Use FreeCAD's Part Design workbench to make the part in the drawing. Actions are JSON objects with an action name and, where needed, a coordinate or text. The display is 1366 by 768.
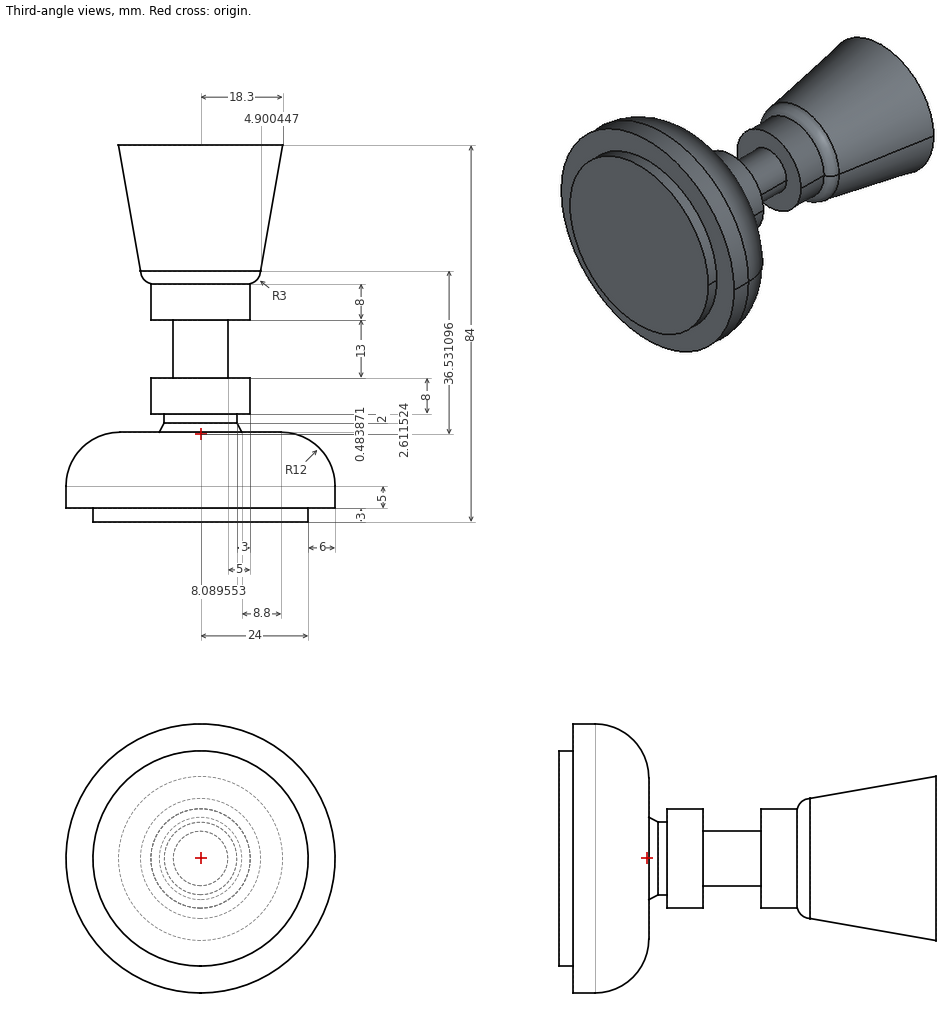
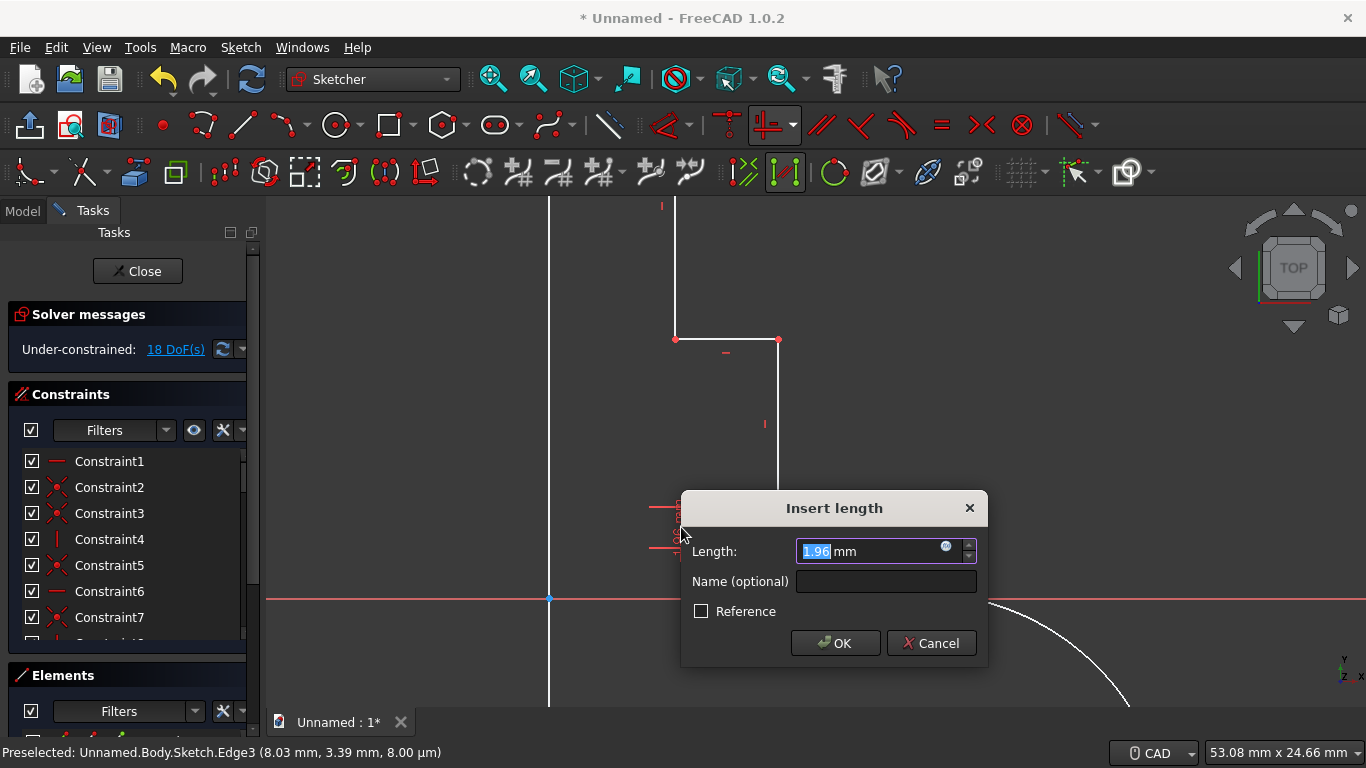
{"action": "type", "text": "2"}
{"action": "key", "text": "Return"}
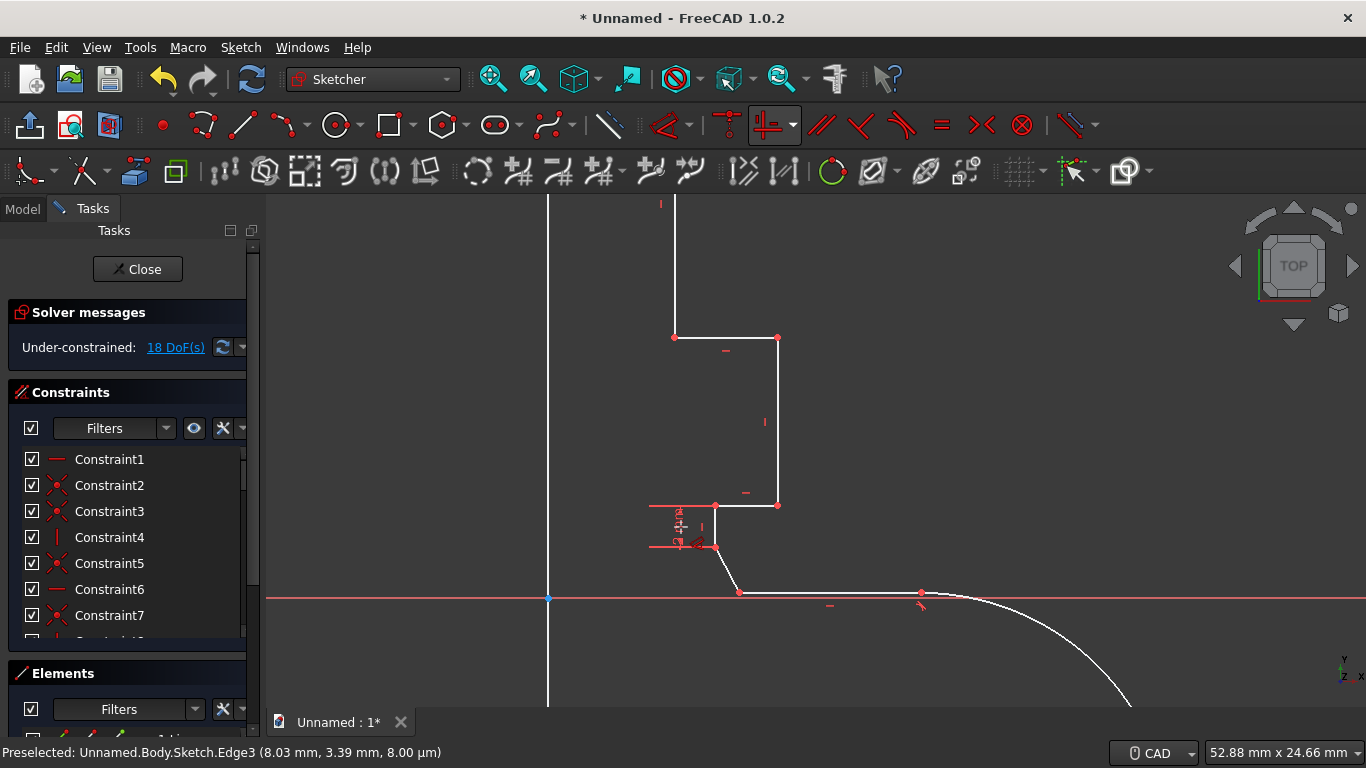
{"action": "left_click", "coordinate": [734, 506]}
{"action": "left_click", "coordinate": [761, 540]}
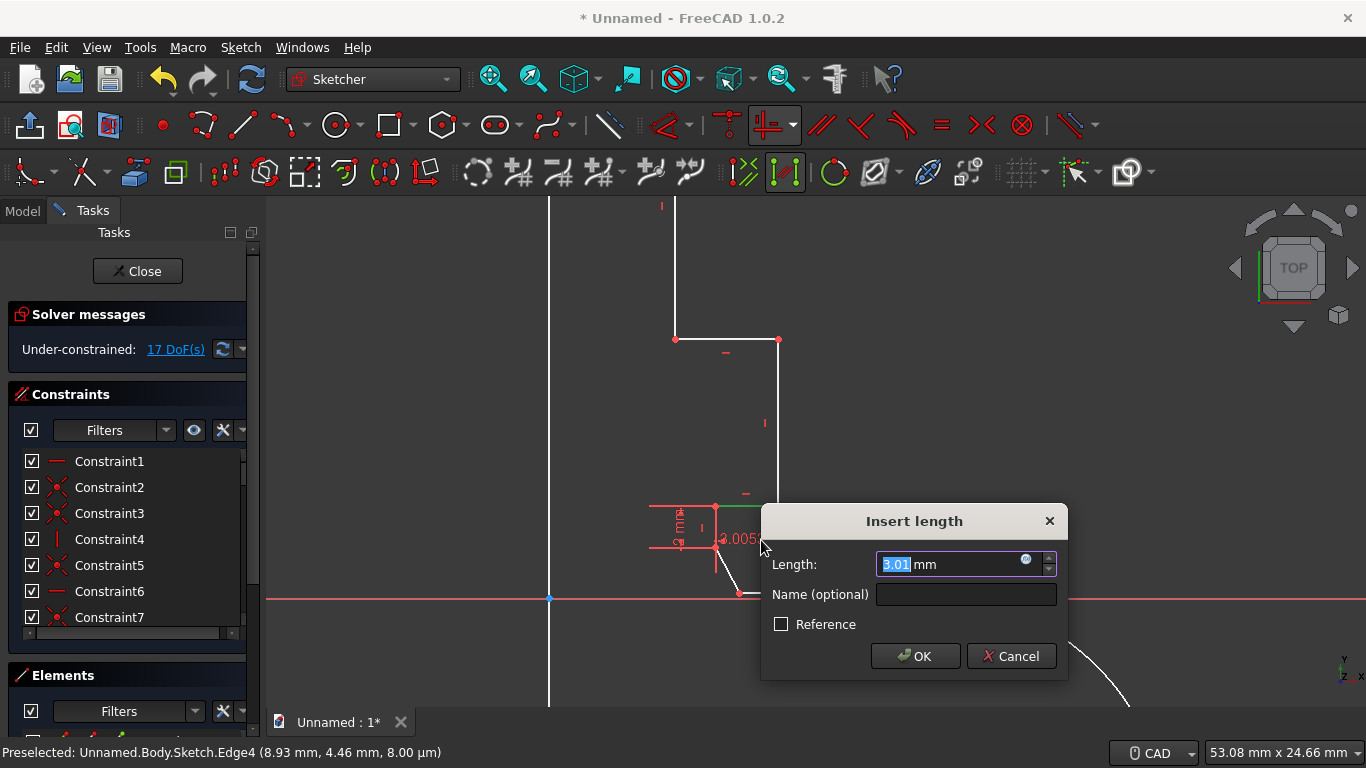
{"action": "type", "text": "3"}
{"action": "key", "text": "Return"}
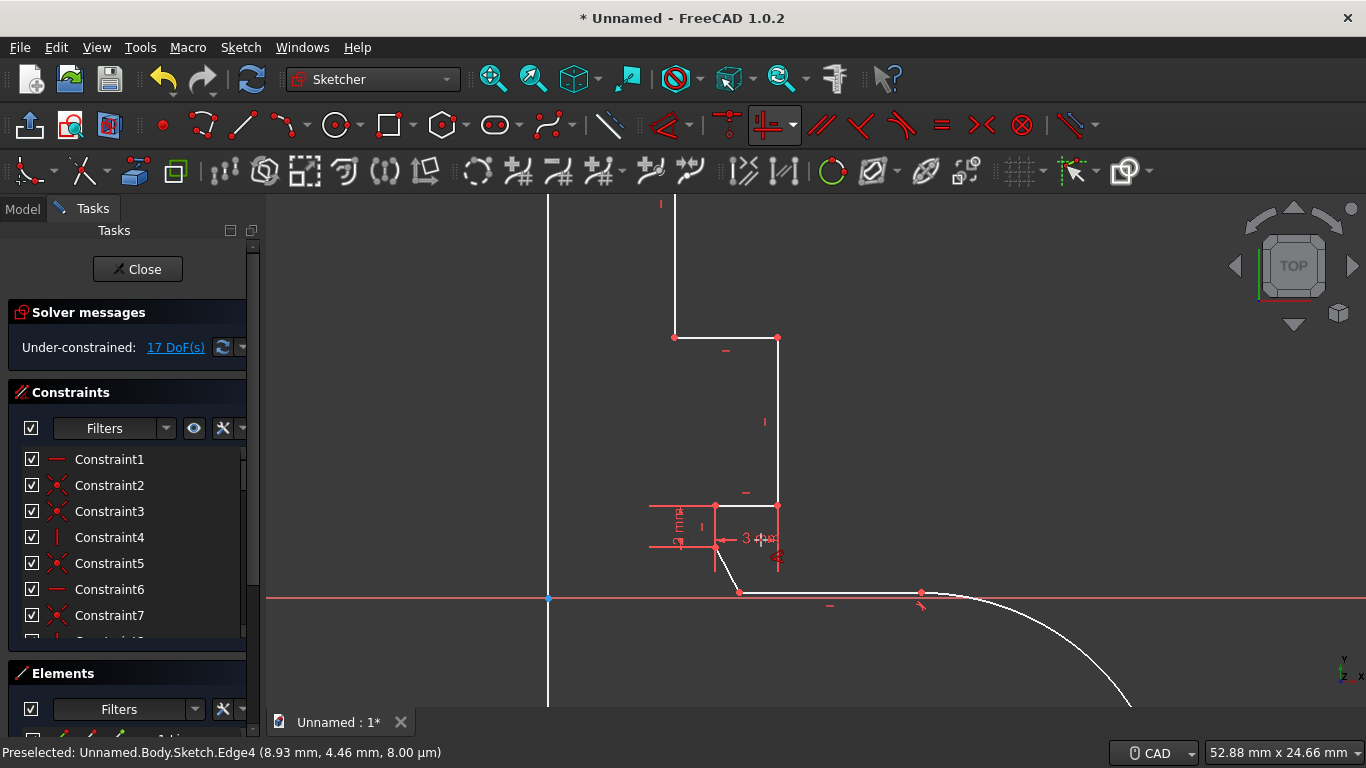
{"action": "scroll", "coordinate": [719, 531], "scroll_direction": "down", "scroll_amount": 8}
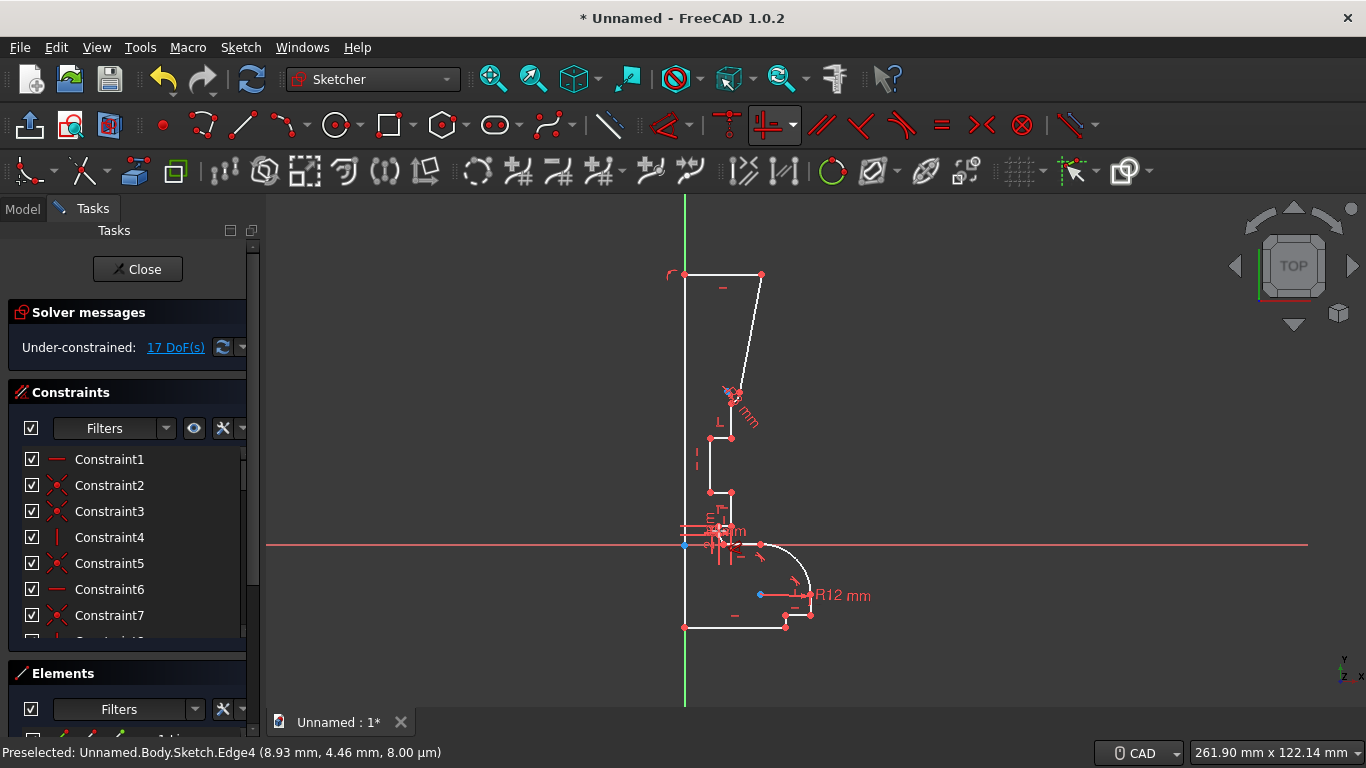
{"action": "scroll", "coordinate": [731, 516], "scroll_direction": "up", "scroll_amount": 2}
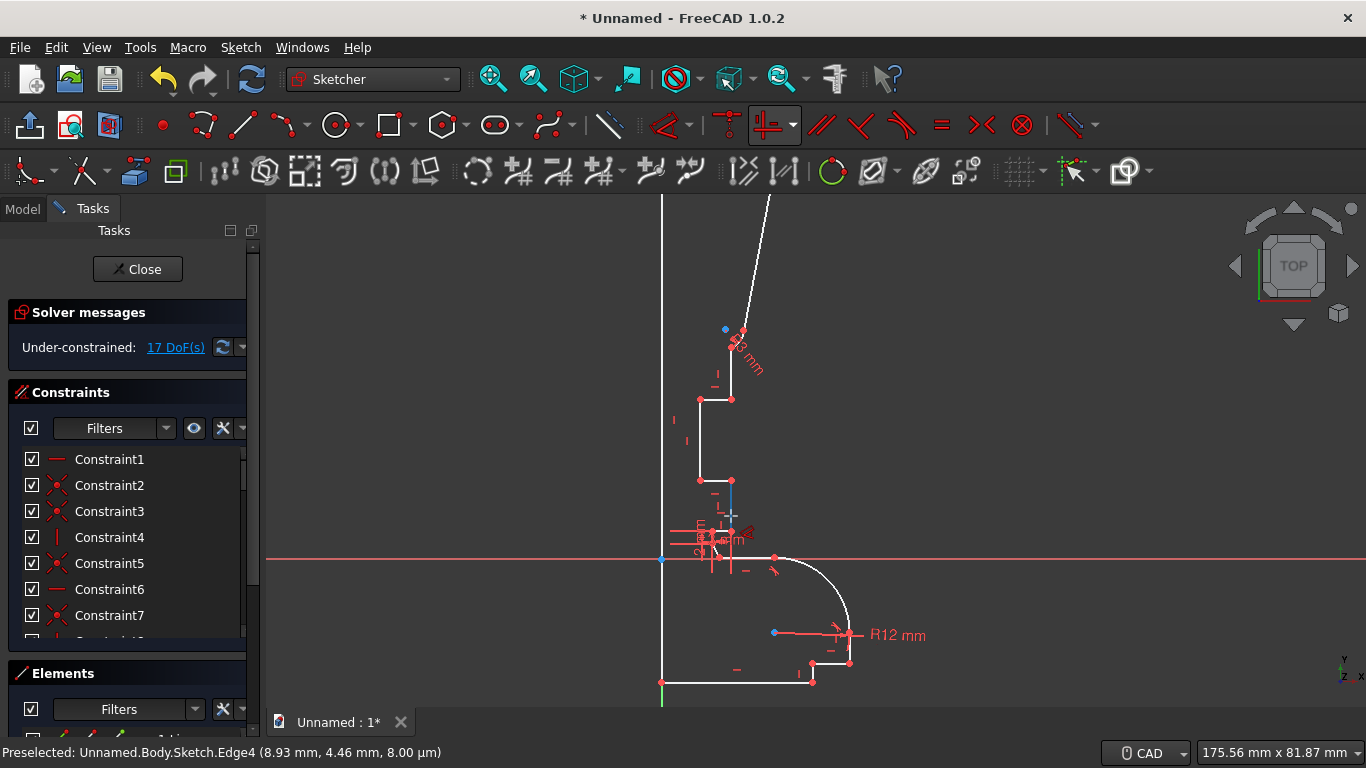
{"action": "left_click", "coordinate": [731, 516]}
{"action": "left_click", "coordinate": [697, 506]}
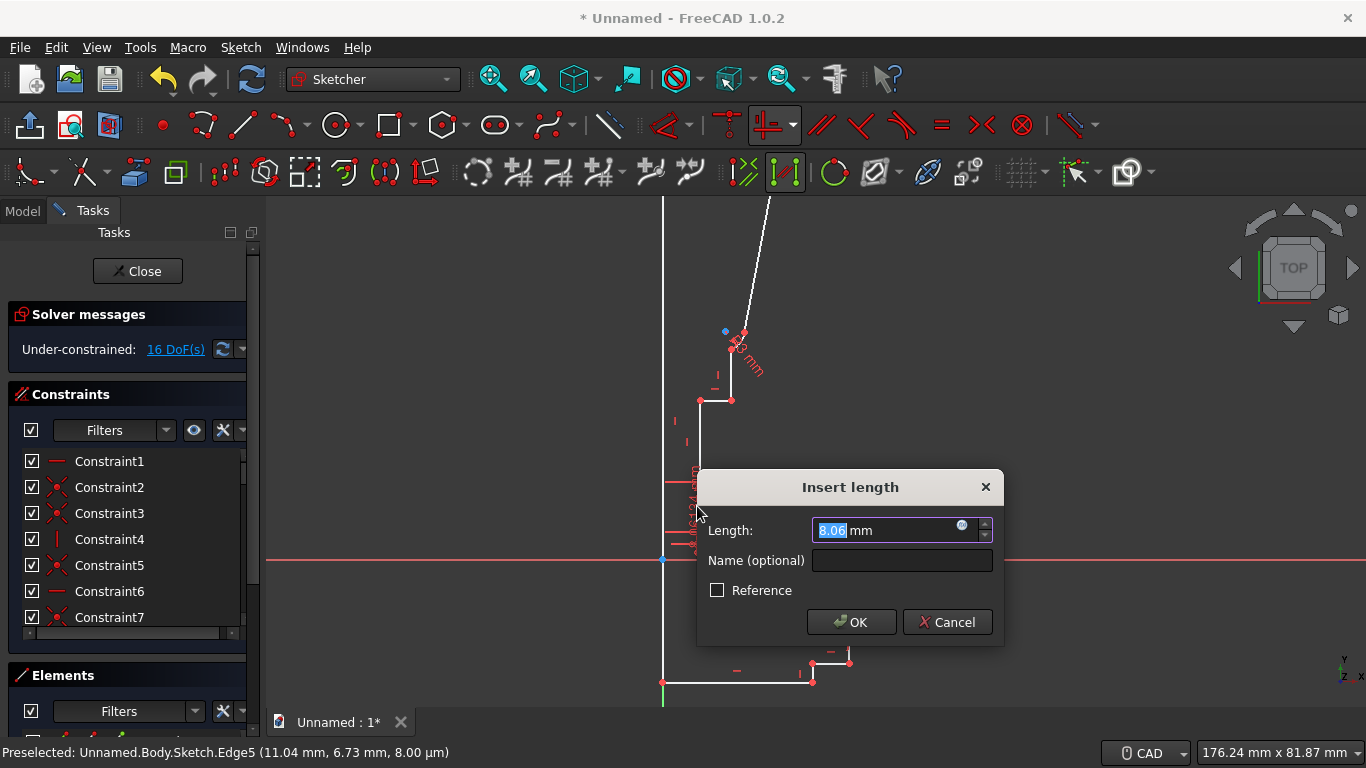
{"action": "type", "text": "8"}
{"action": "key", "text": "Return"}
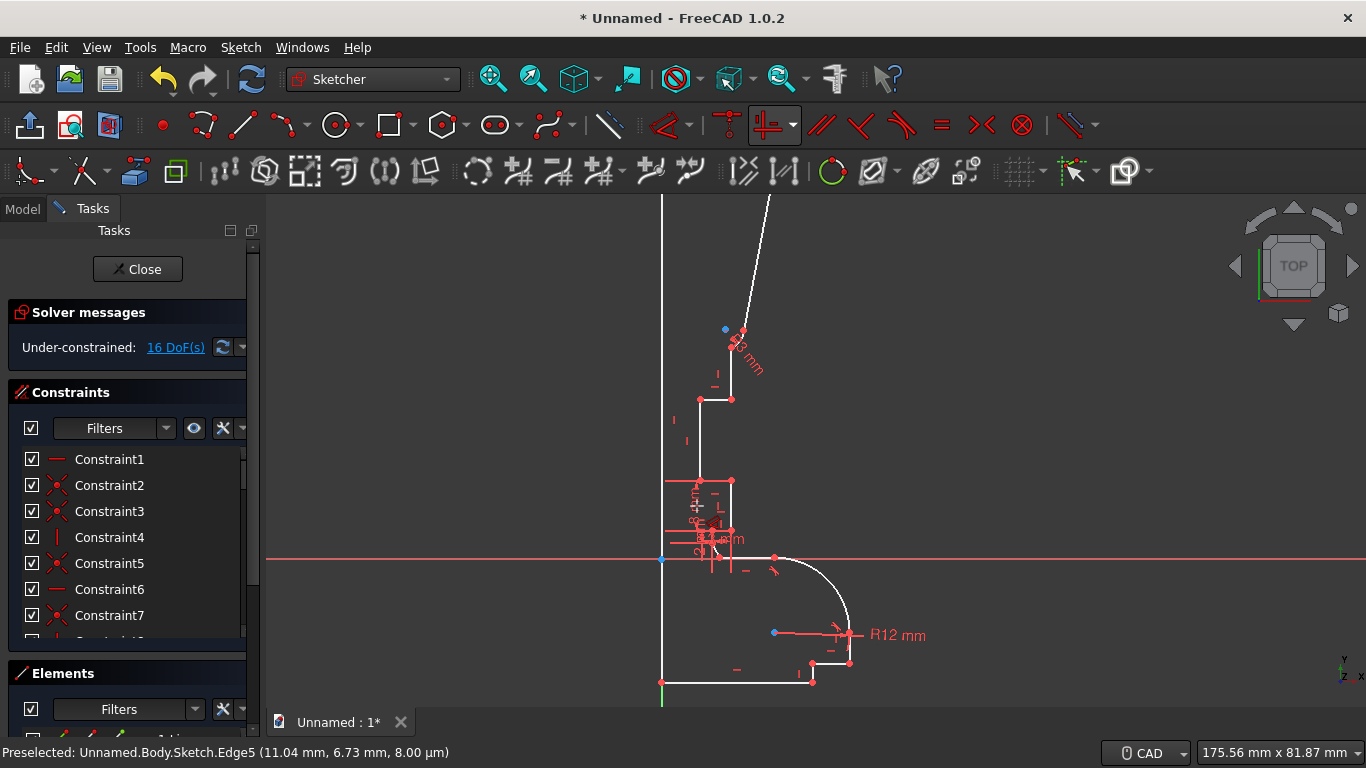
{"action": "scroll", "coordinate": [722, 481], "scroll_direction": "up", "scroll_amount": 2}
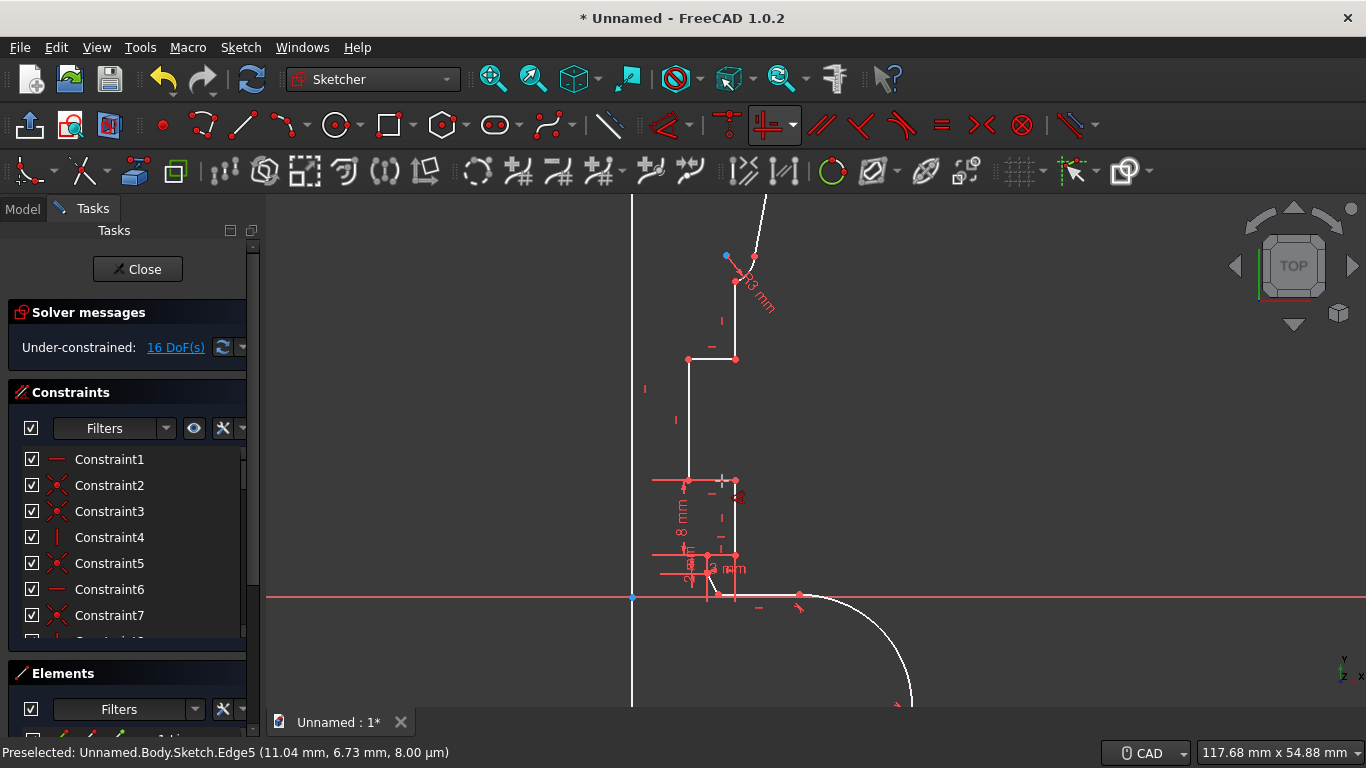
{"action": "left_click", "coordinate": [721, 480]}
{"action": "left_click", "coordinate": [712, 446]}